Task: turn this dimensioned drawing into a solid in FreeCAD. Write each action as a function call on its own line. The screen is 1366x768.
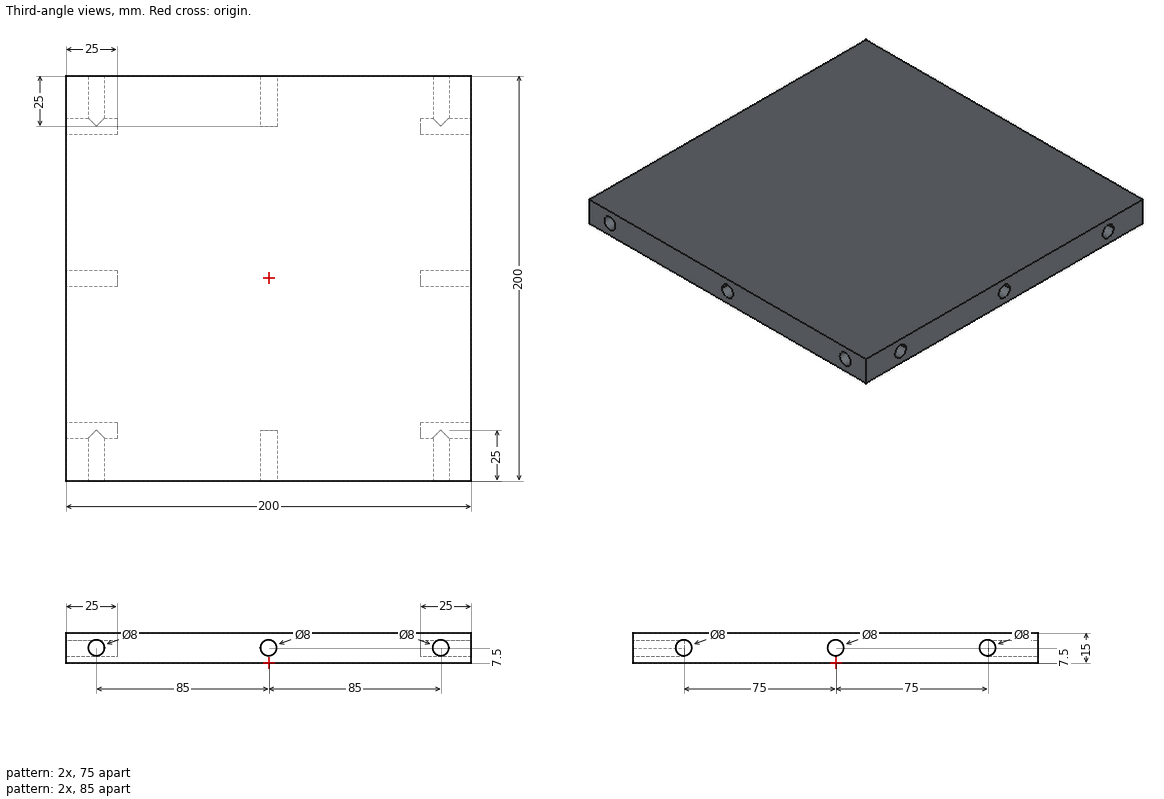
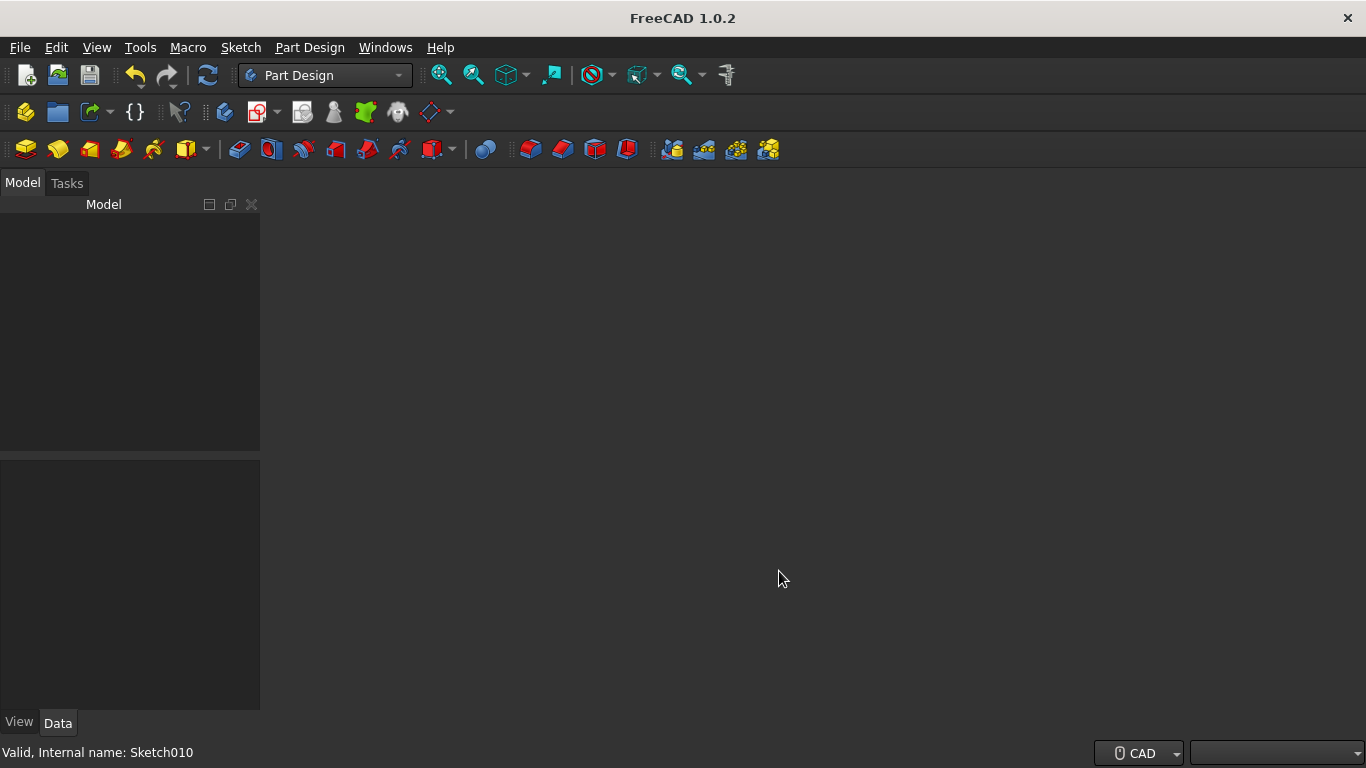
click(26, 76)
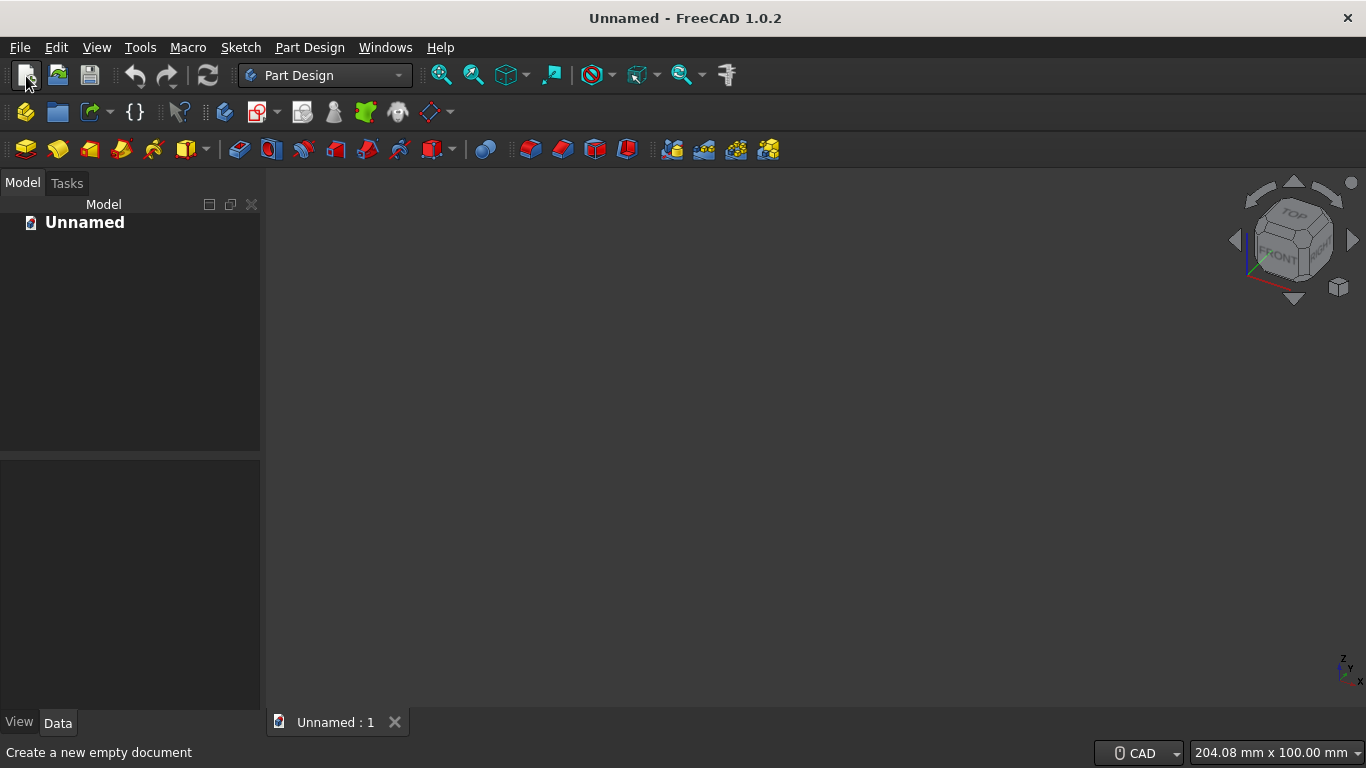
click(258, 112)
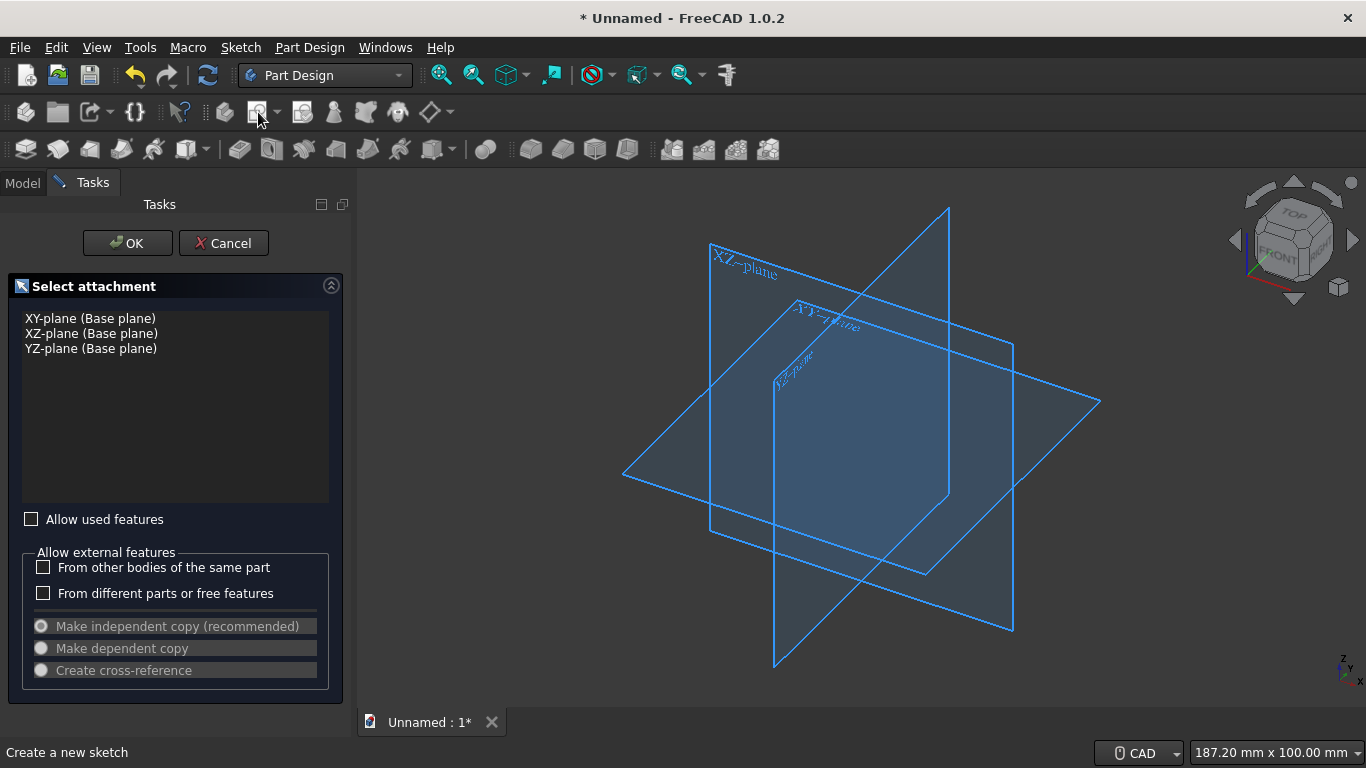
click(82, 318)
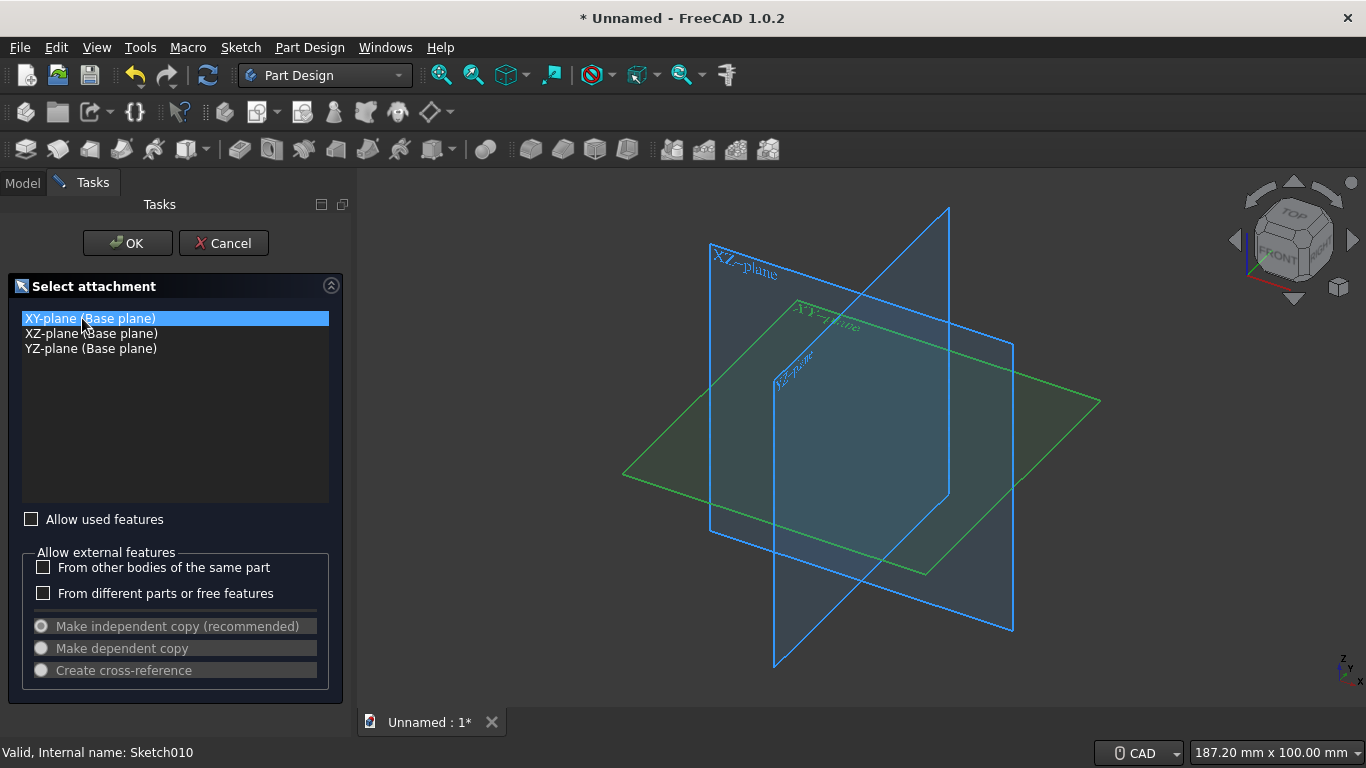
click(128, 243)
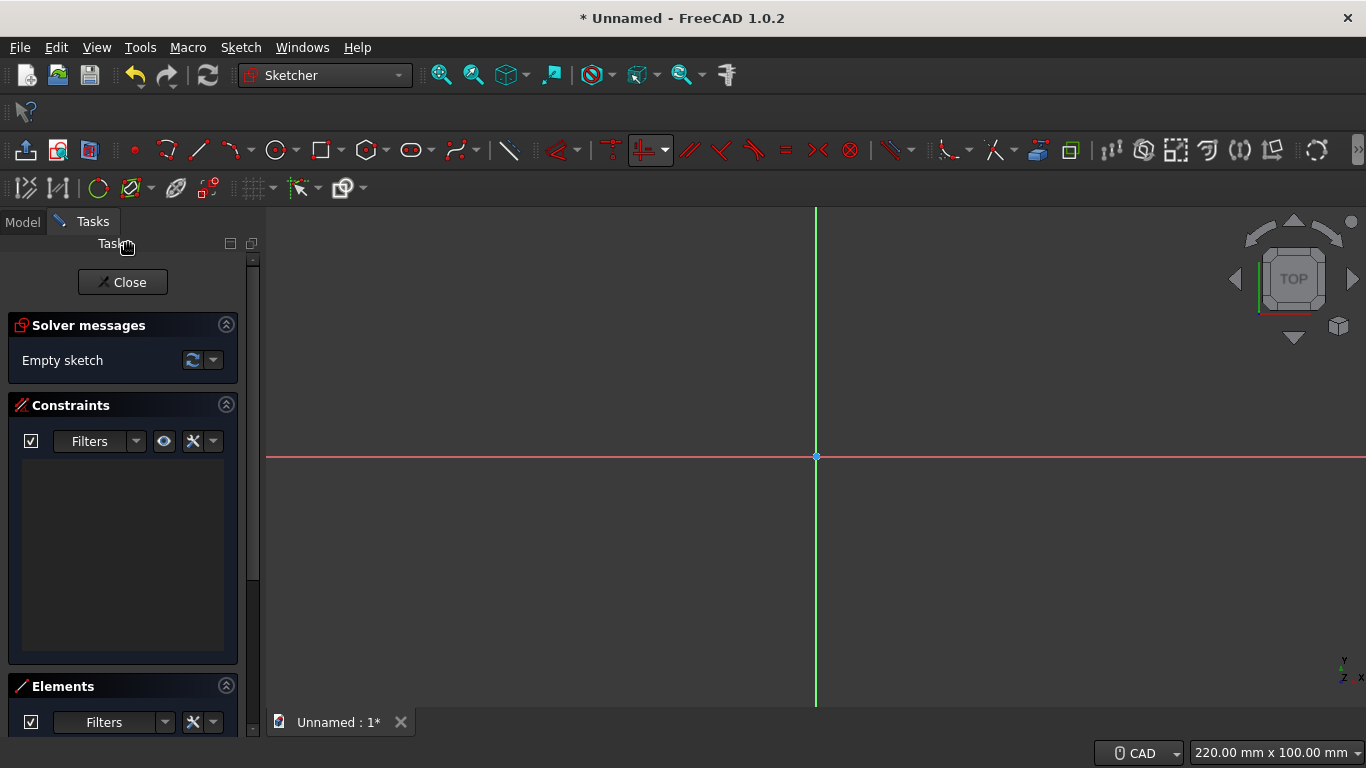
scroll(718, 457, down, 6)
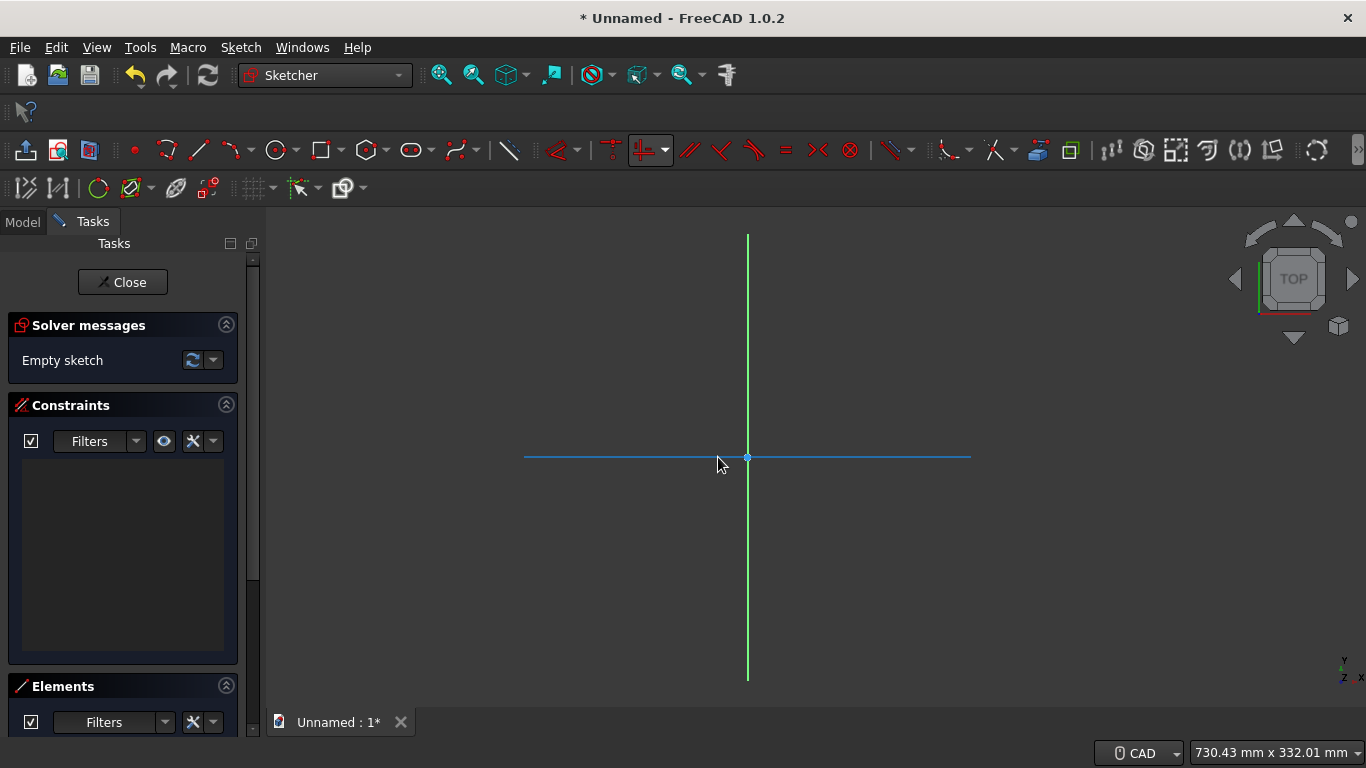
key(g)
key(v)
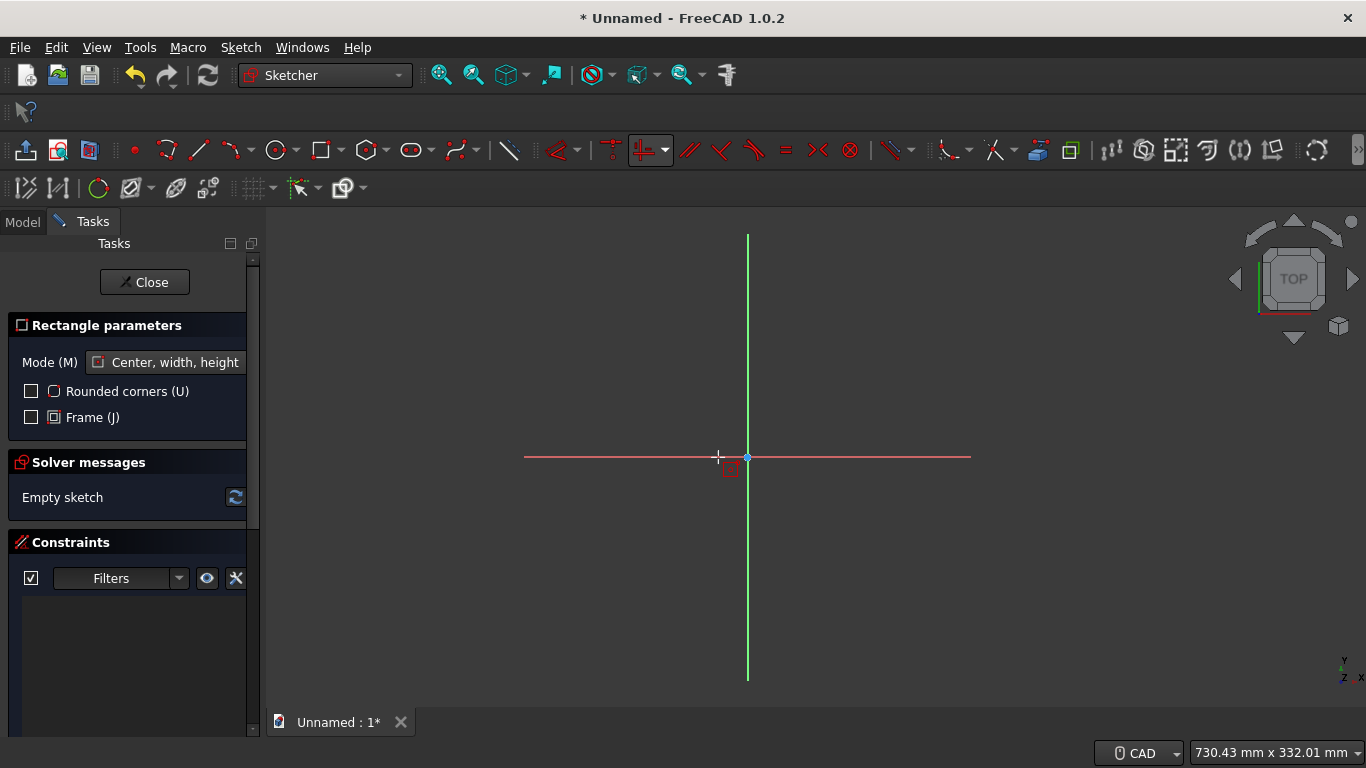
click(748, 457)
move(898, 307)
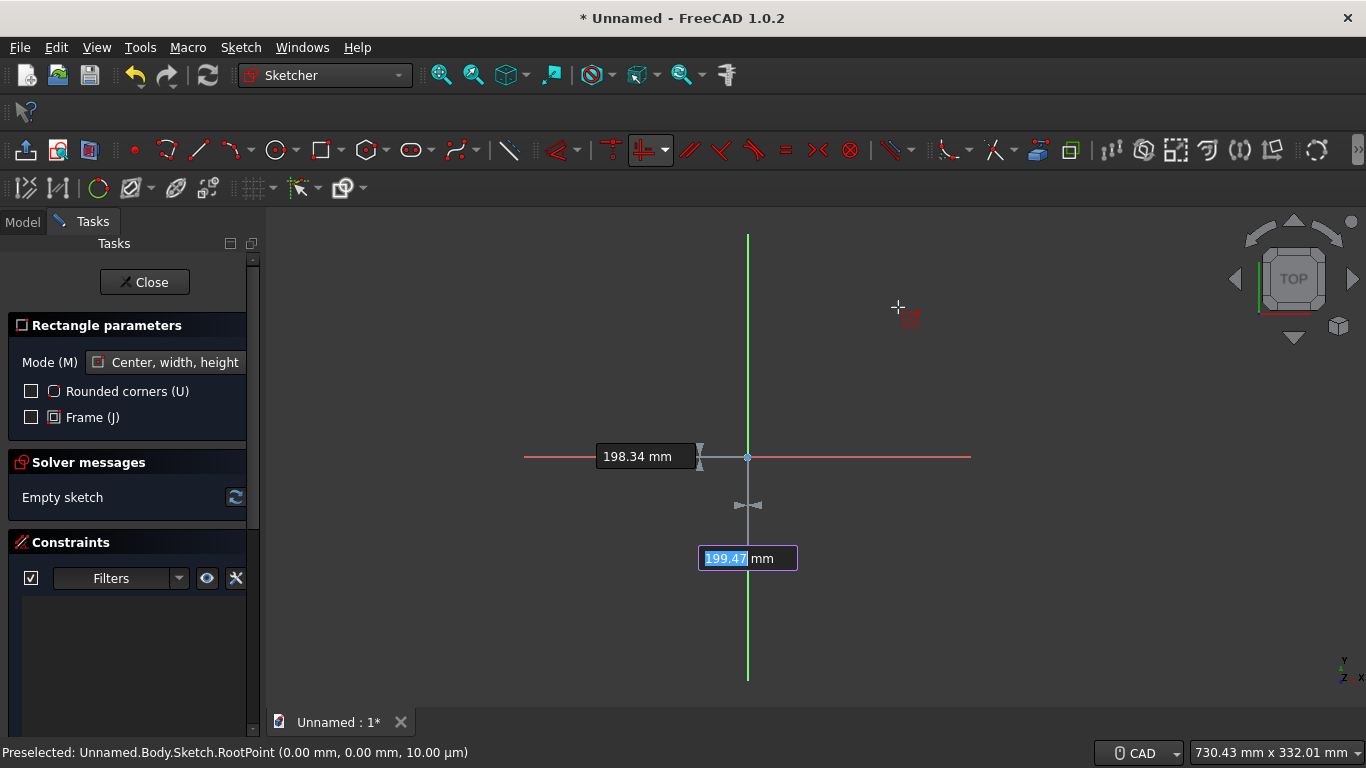
text(200)
key(Tab)
text(200)
key(Return)
key(Escape)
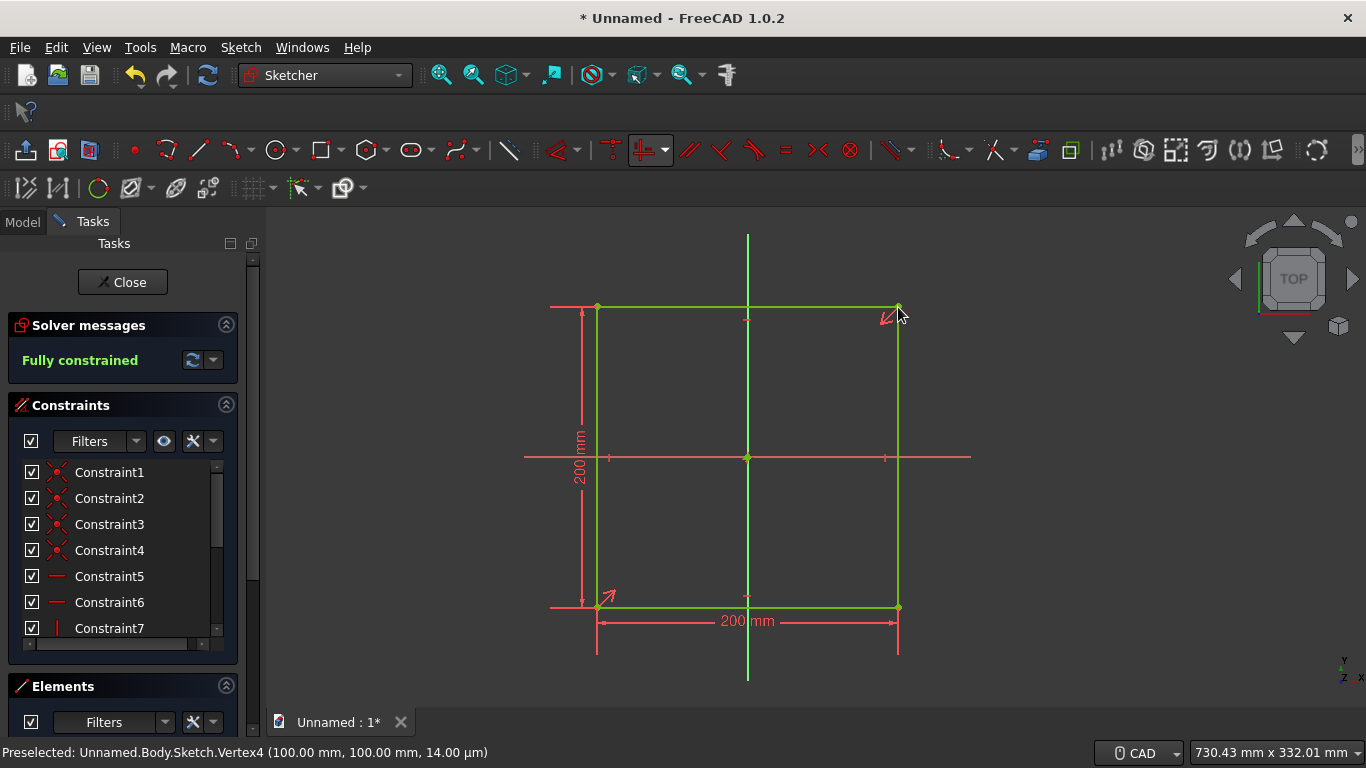
click(123, 282)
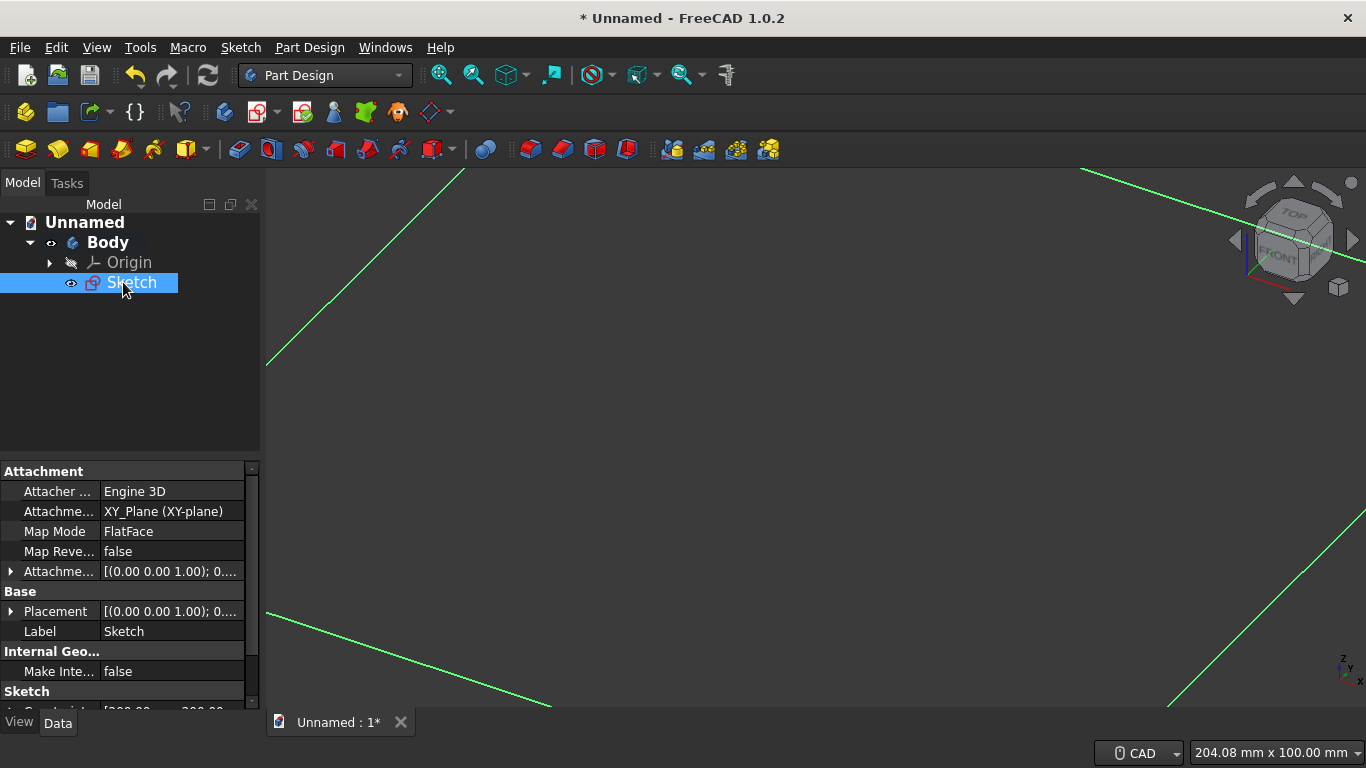
click(26, 150)